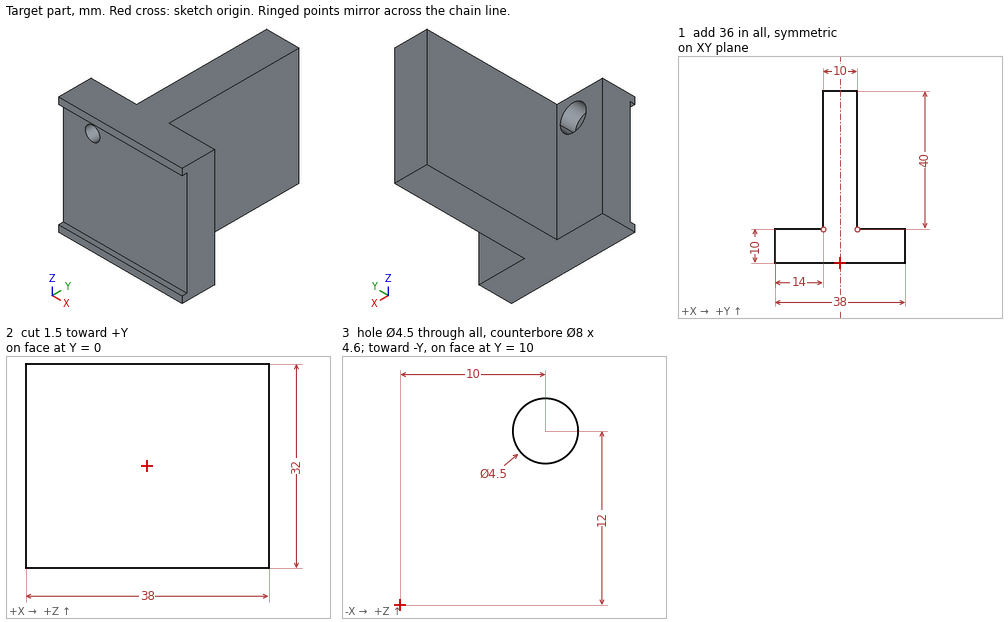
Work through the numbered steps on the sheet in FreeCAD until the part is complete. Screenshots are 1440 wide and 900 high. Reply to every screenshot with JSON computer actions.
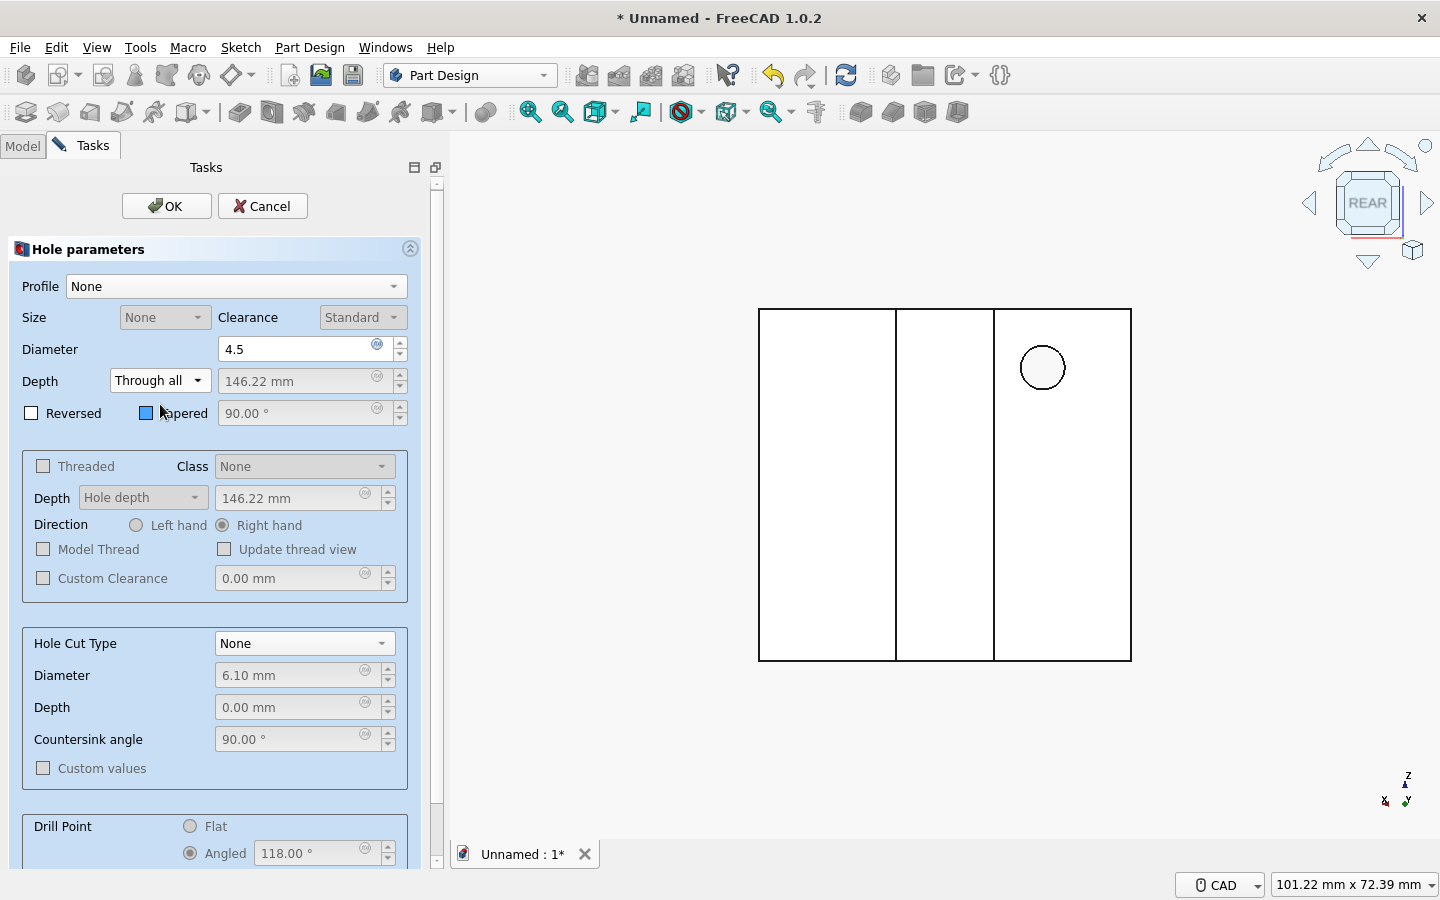
{"action": "left_click", "coordinate": [306, 644]}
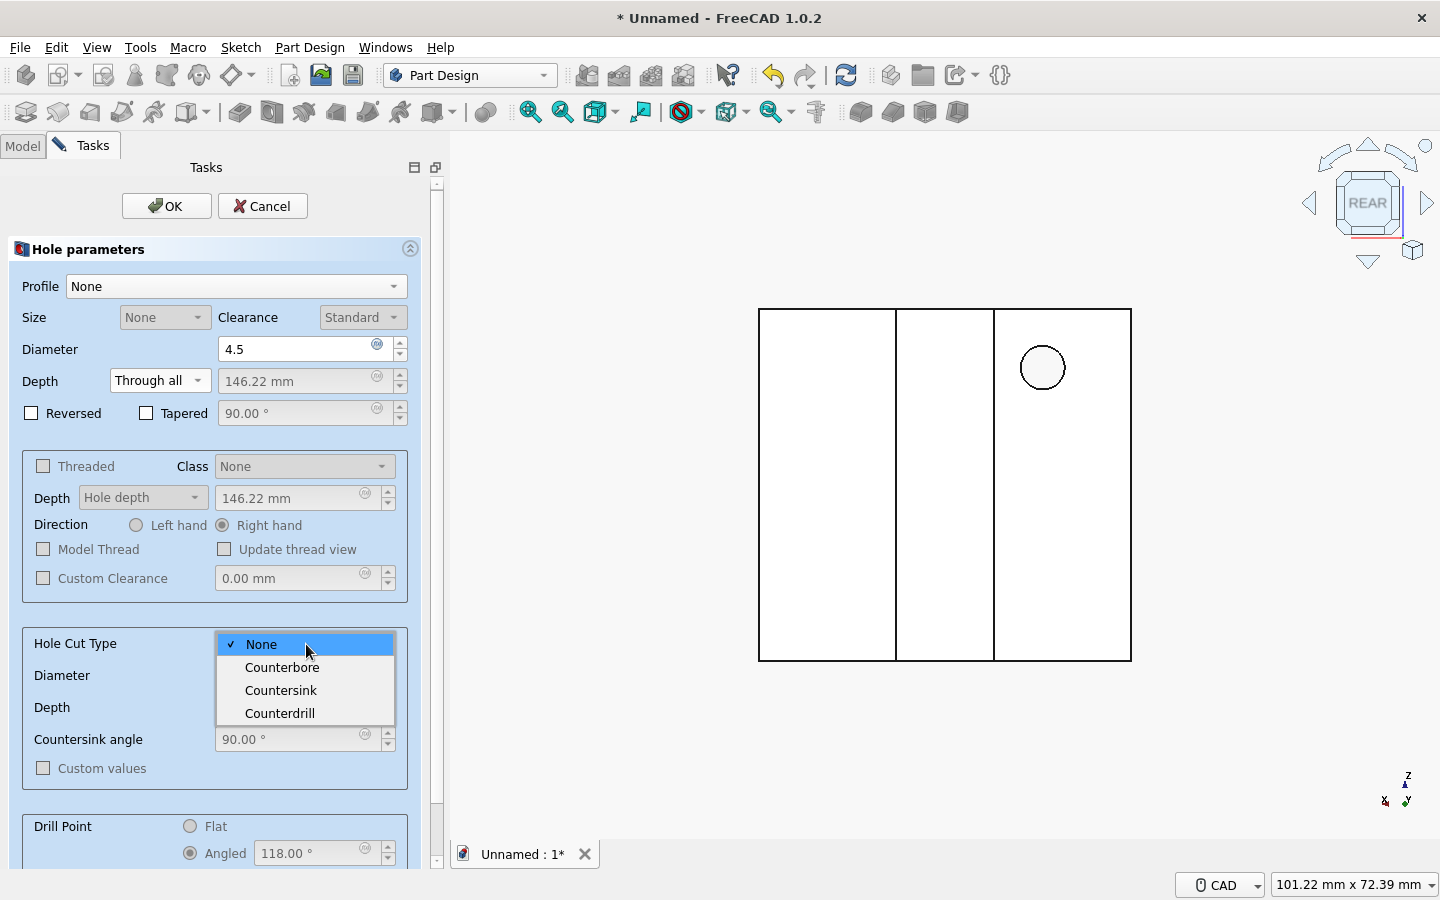
{"action": "left_click", "coordinate": [304, 668]}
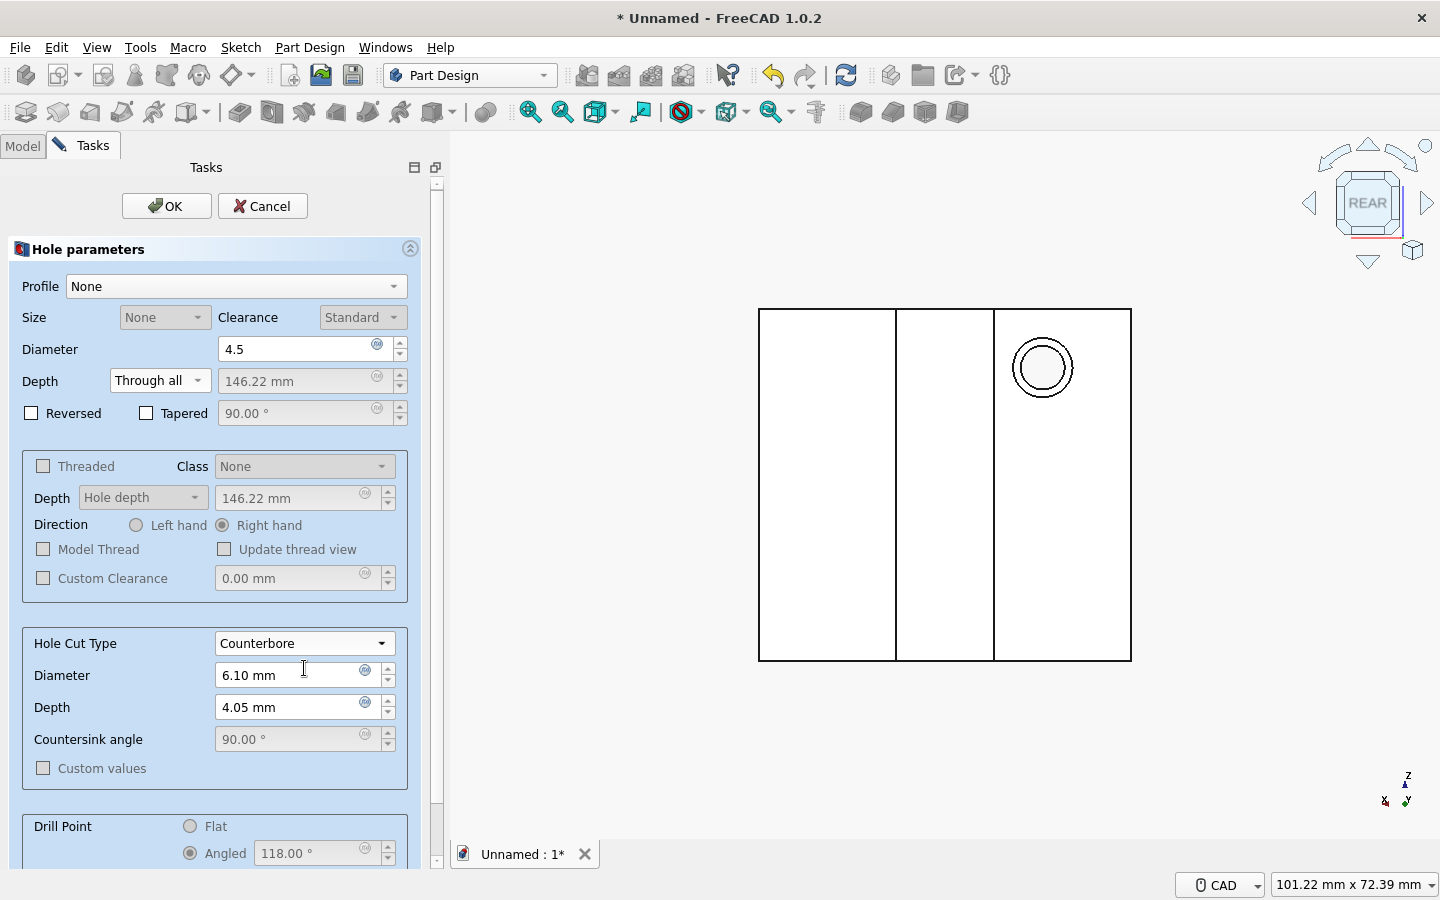
{"action": "triple_click", "coordinate": [298, 675]}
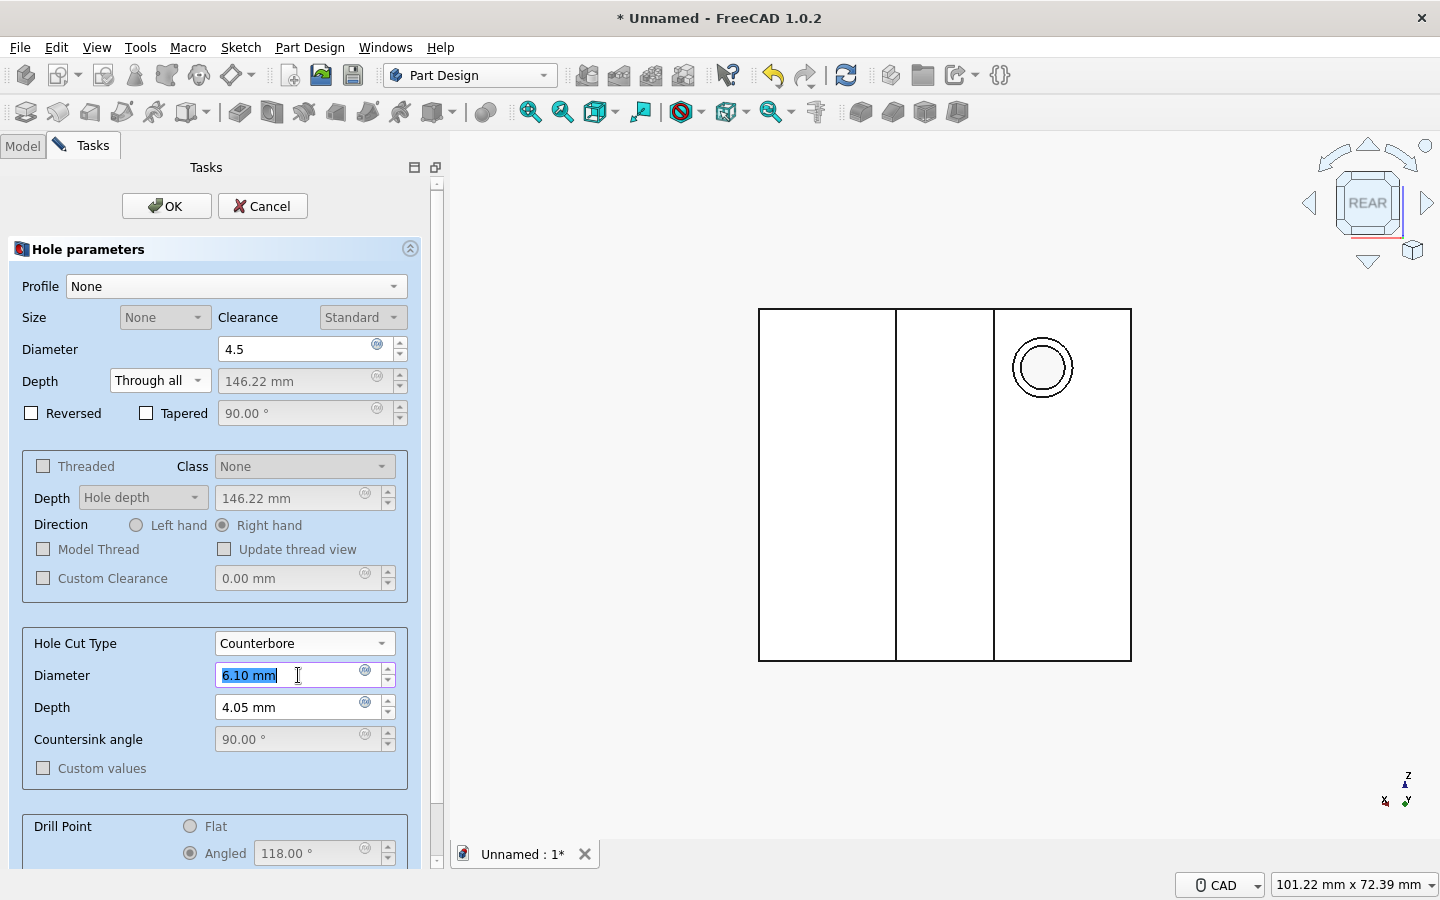
{"action": "type", "text": "8"}
{"action": "key", "text": "Tab"}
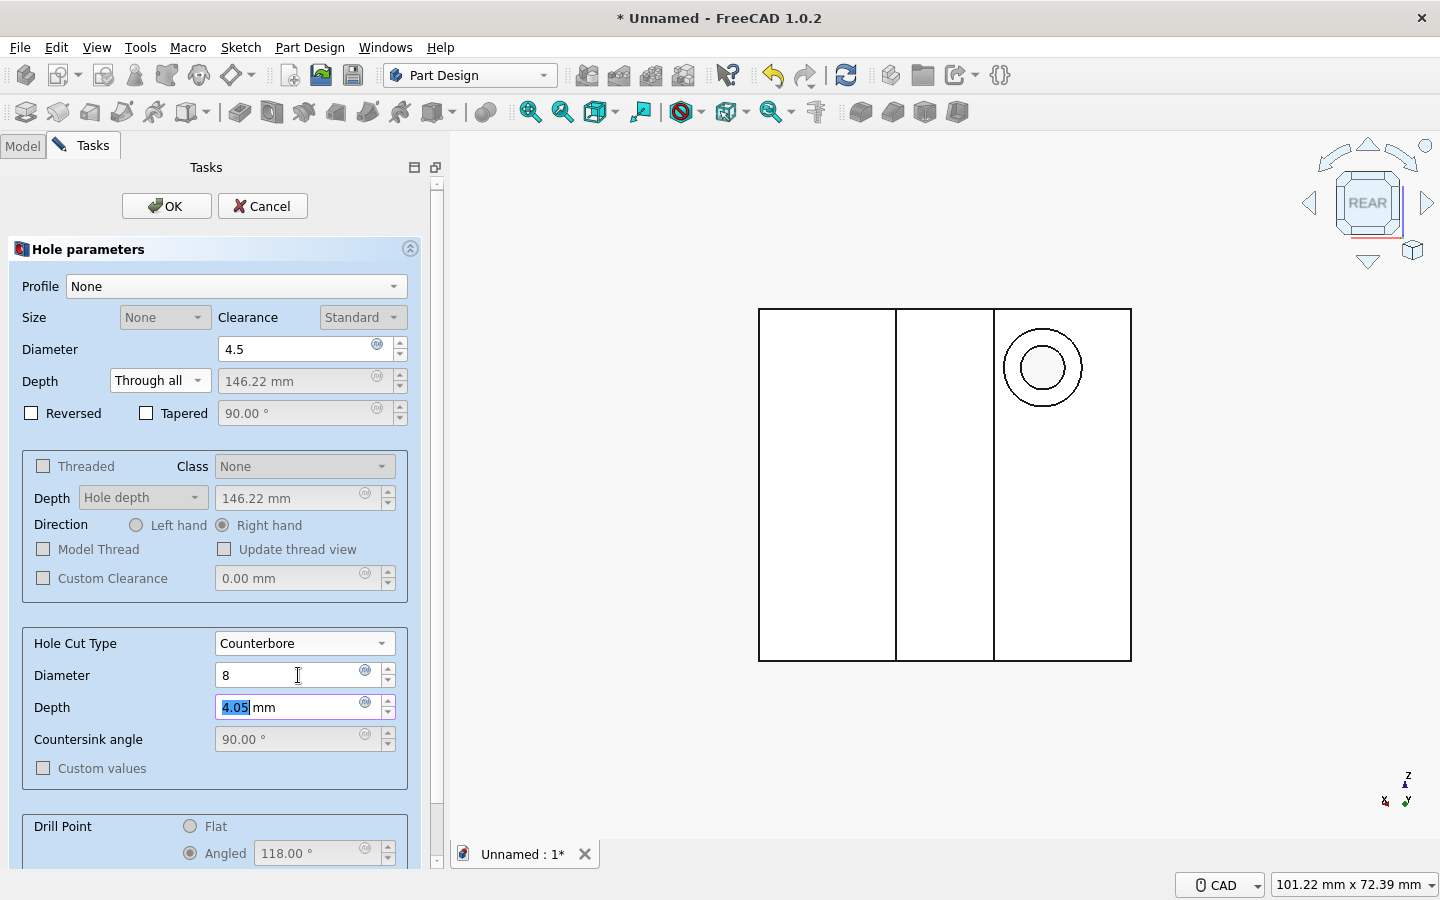
{"action": "type", "text": "4.6"}
{"action": "key", "text": "Tab"}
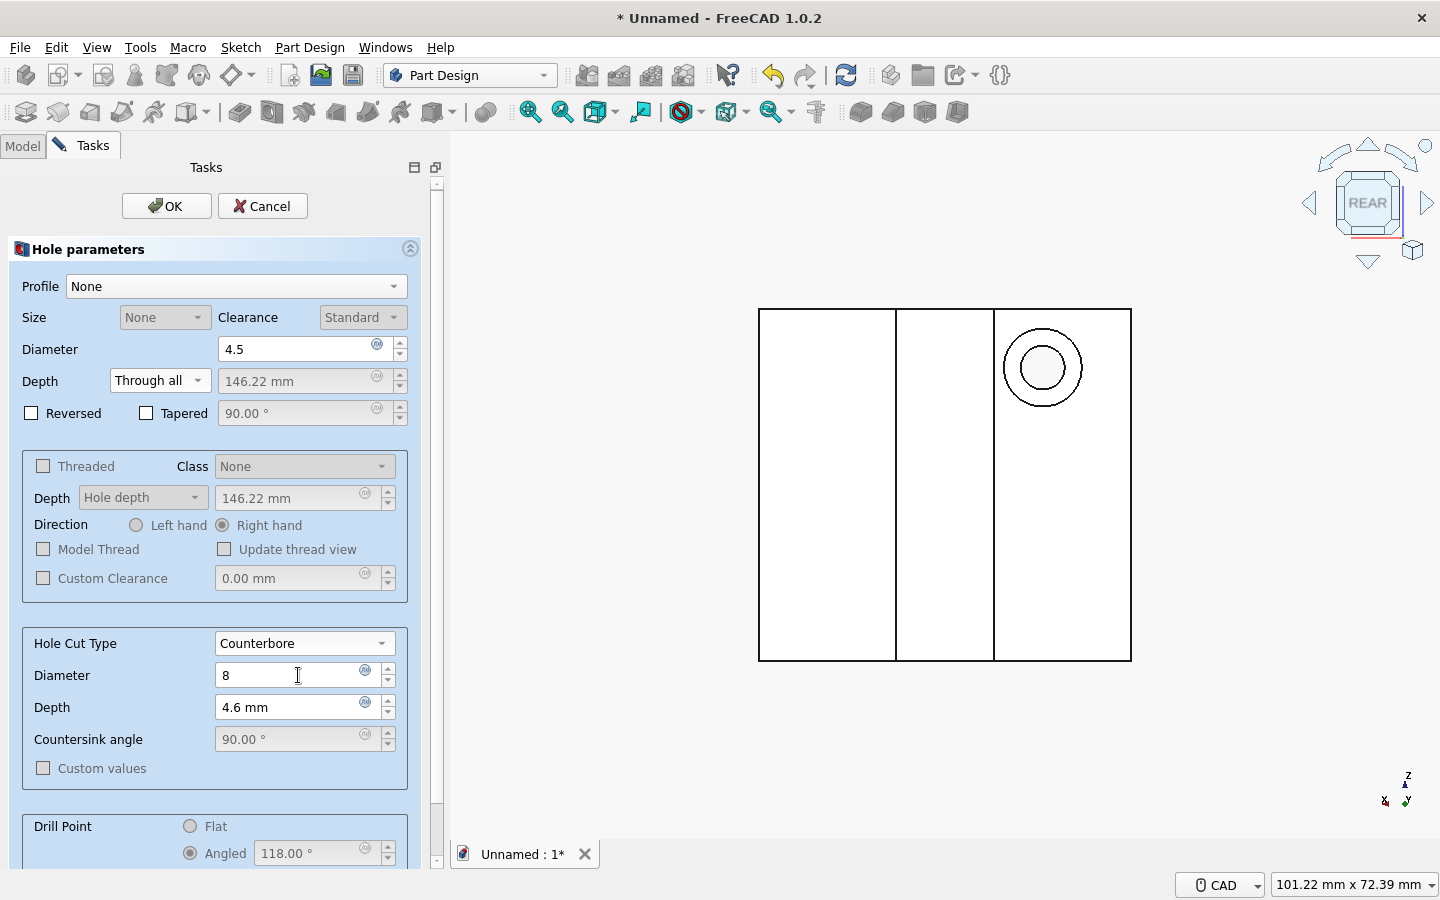
{"action": "left_click", "coordinate": [167, 206]}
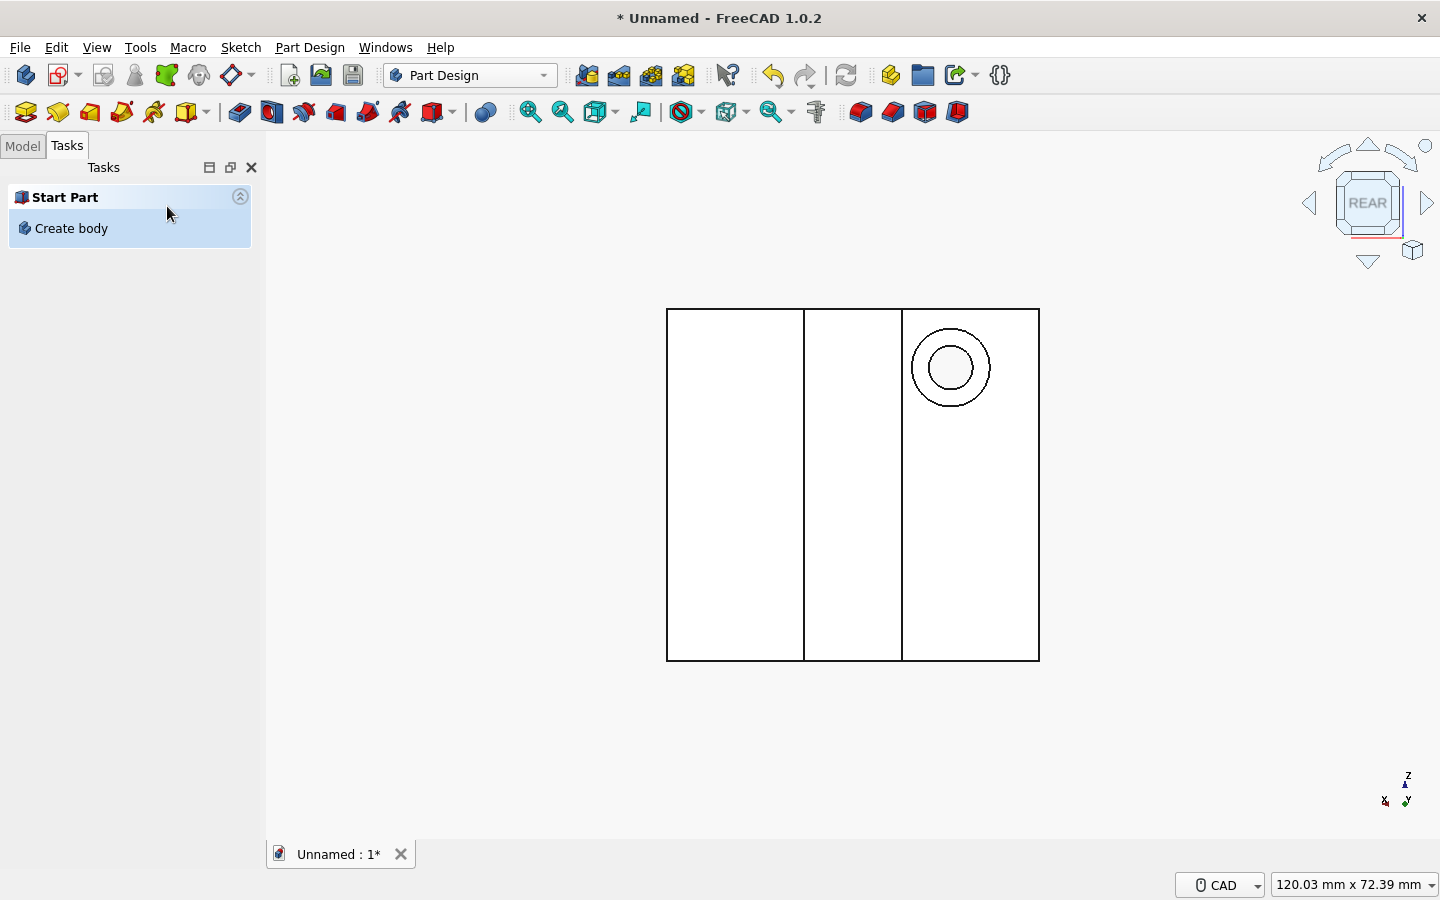
{"action": "key", "text": "0"}